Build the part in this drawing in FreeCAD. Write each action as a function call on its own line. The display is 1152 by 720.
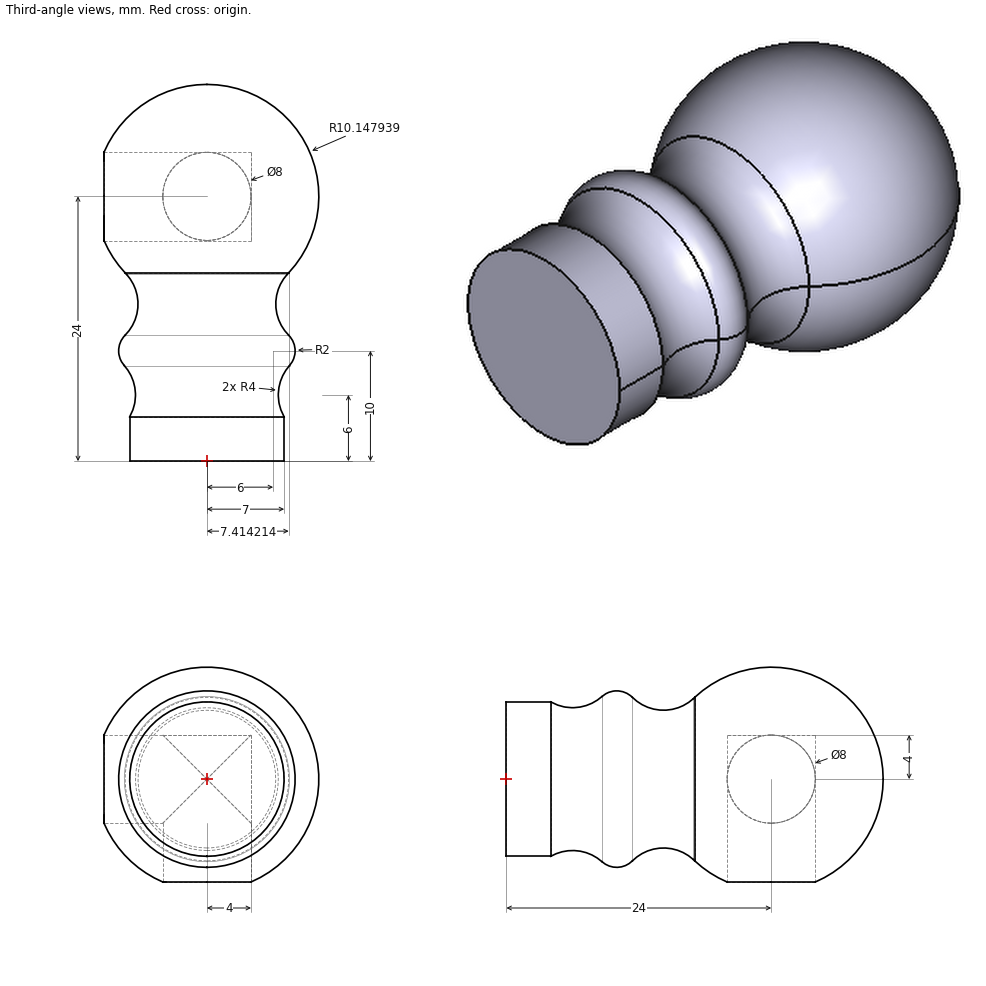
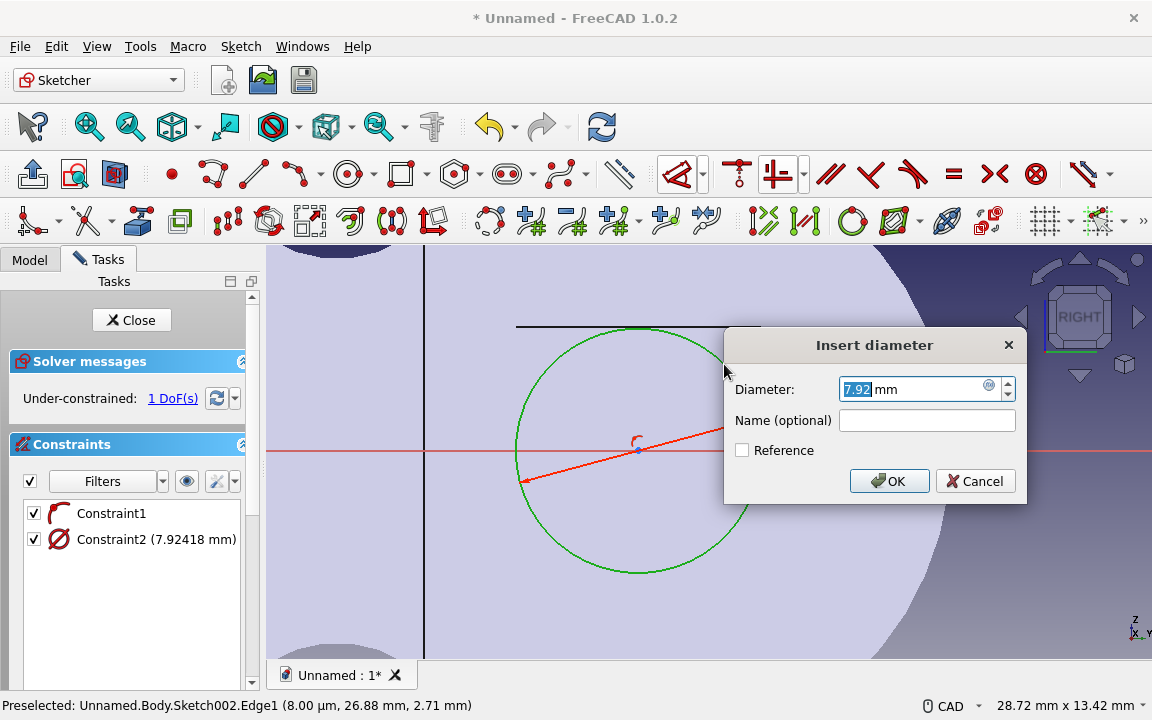
text(8)
key(Return)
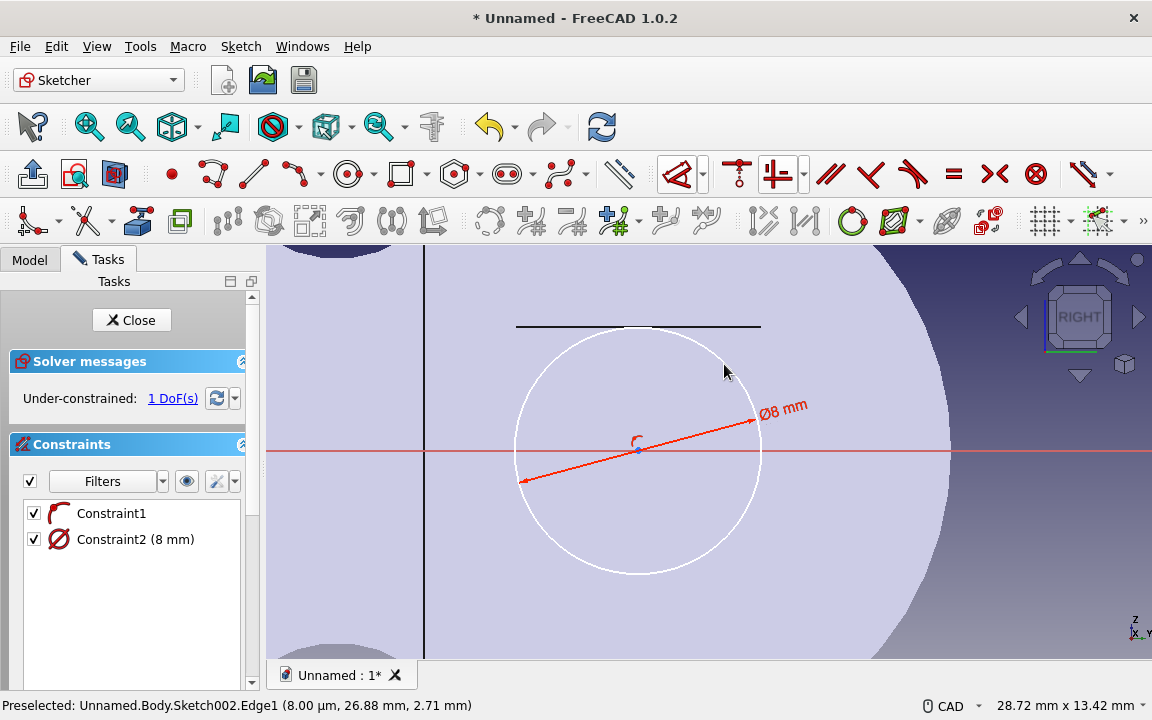
click(638, 451)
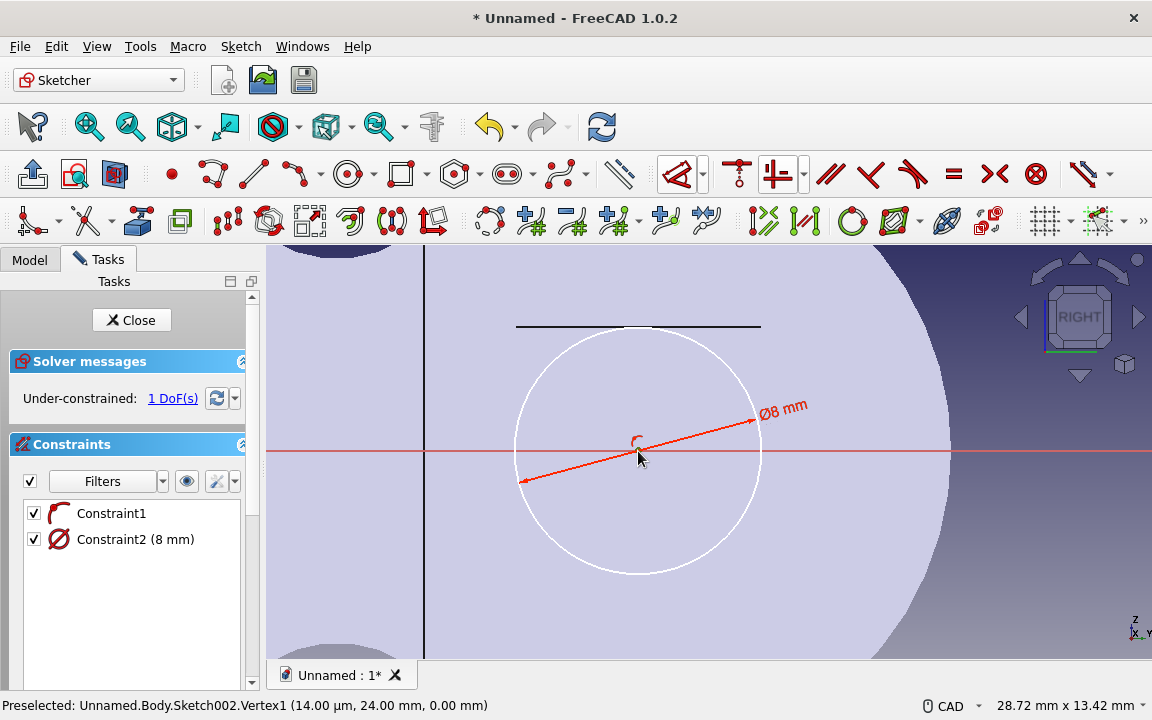
key(l)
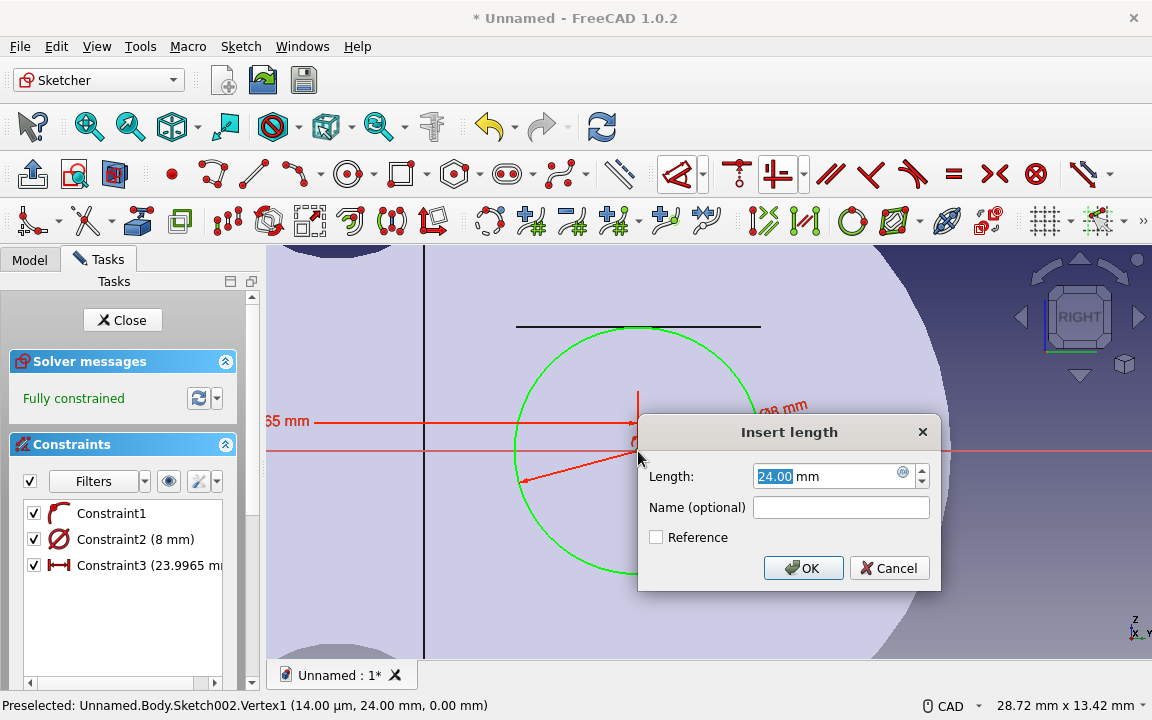
text(24)
key(Return)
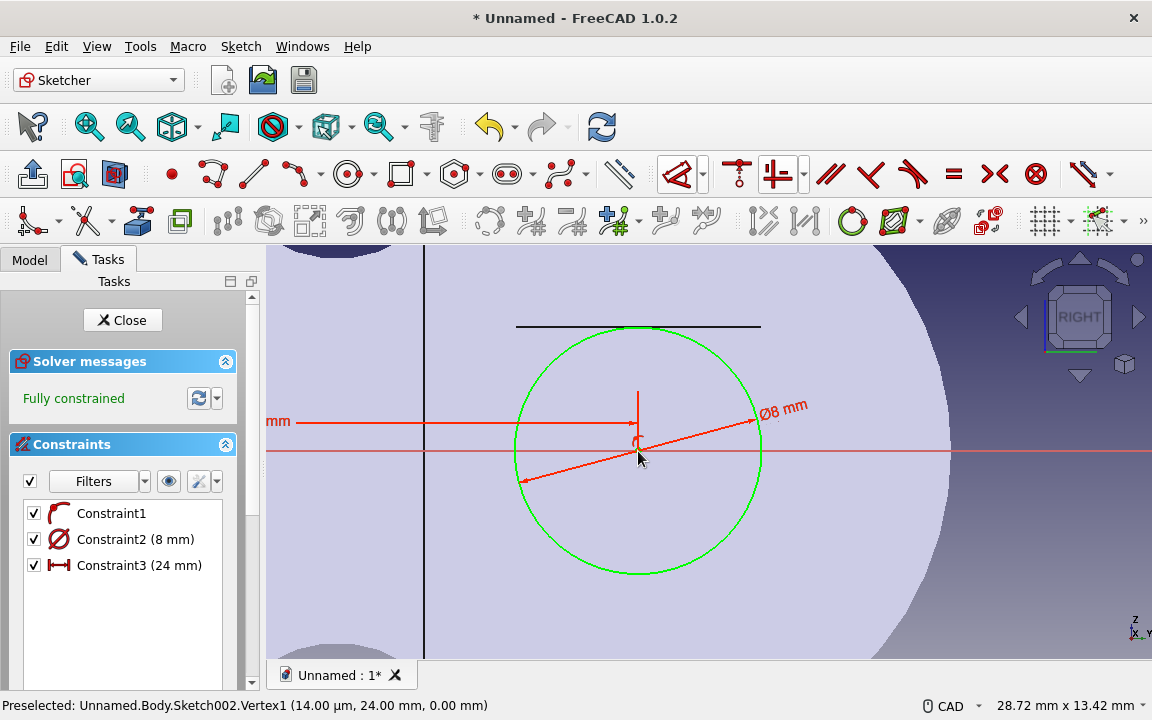
click(123, 320)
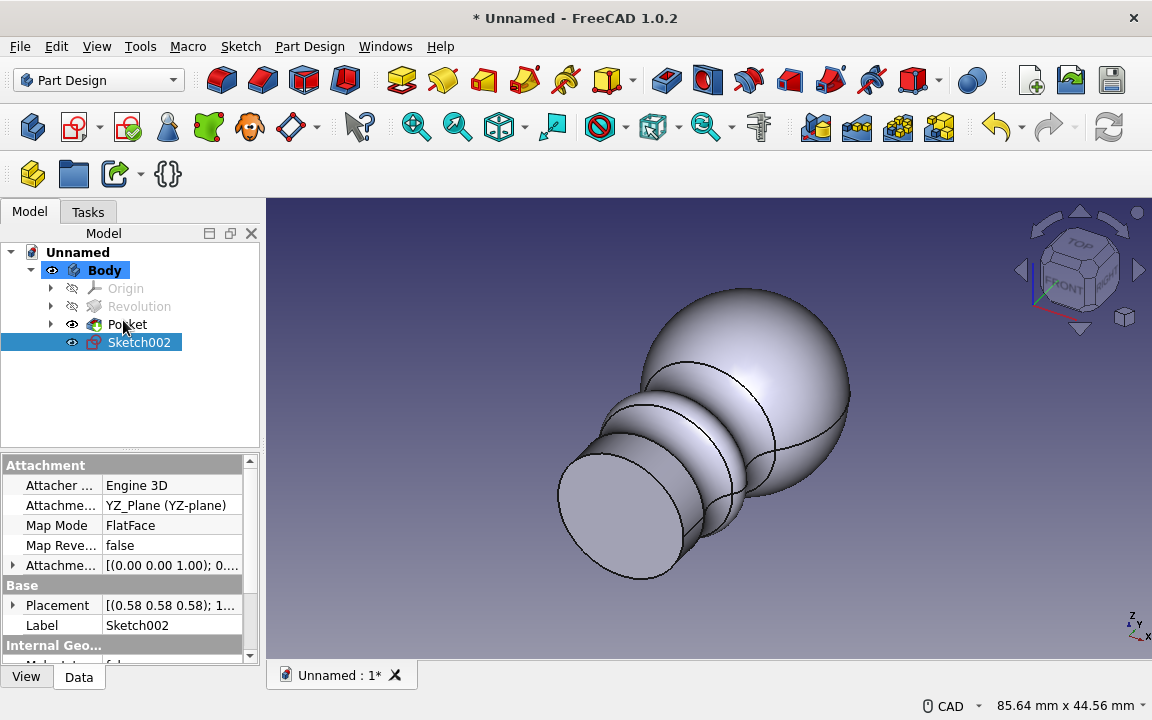
click(667, 80)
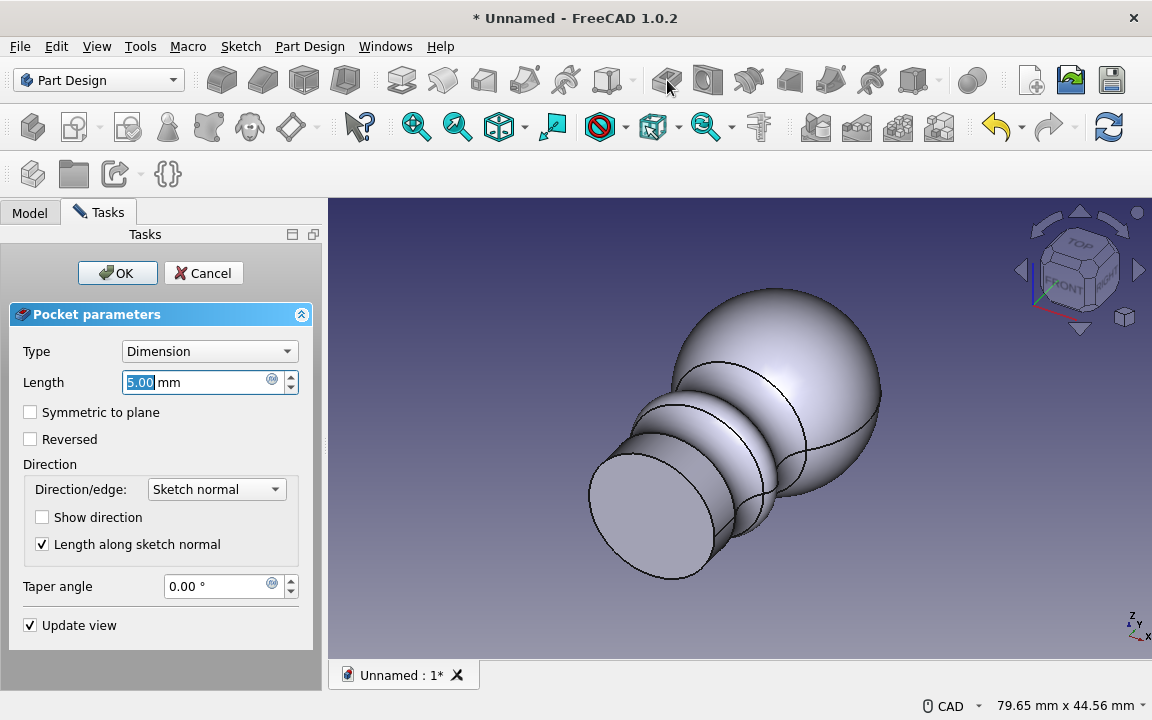
click(210, 352)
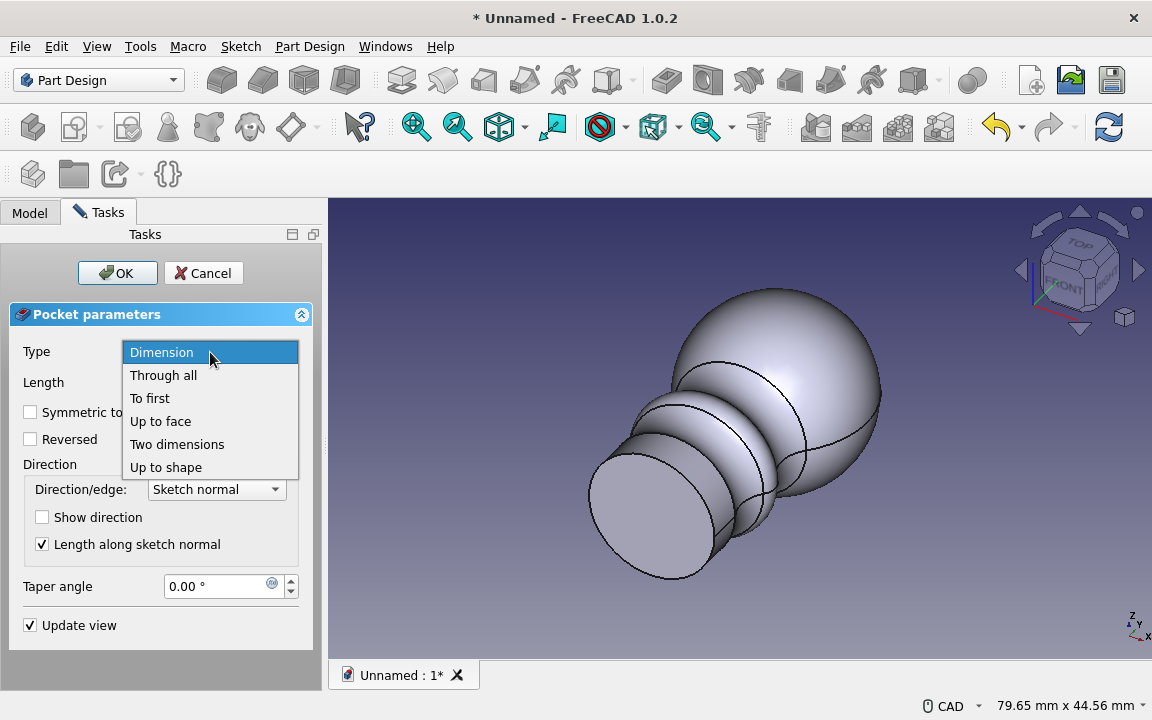
click(208, 444)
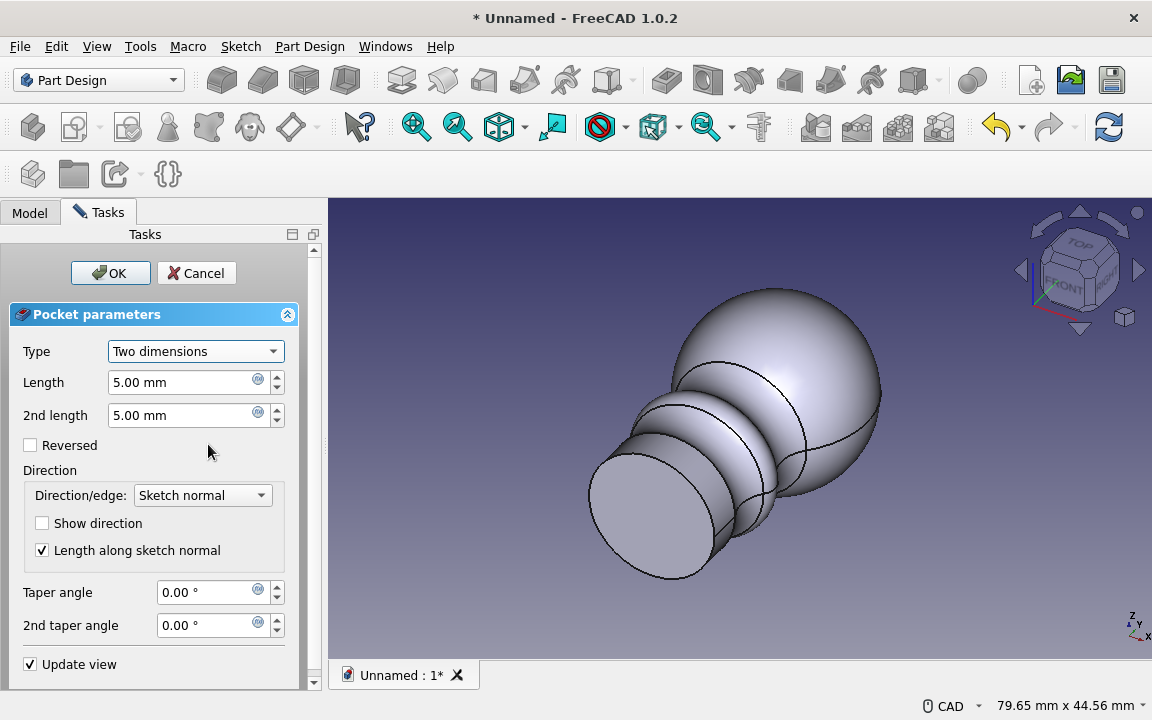
triple_click(190, 382)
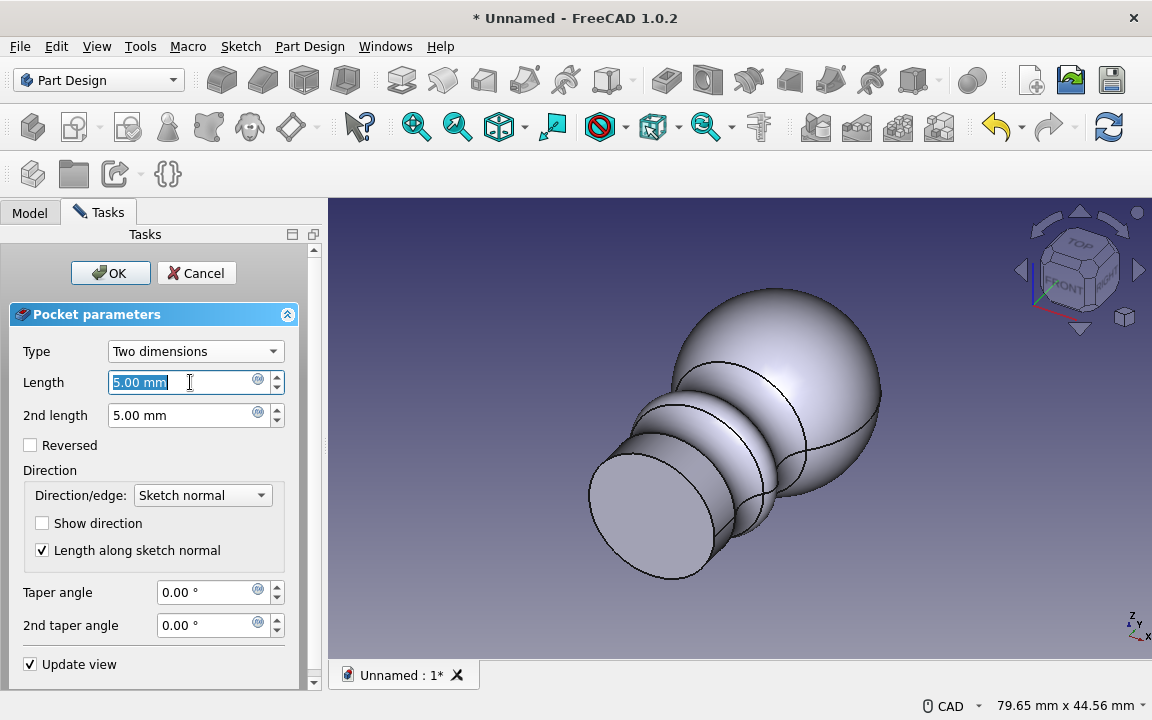
text(4)
key(Tab)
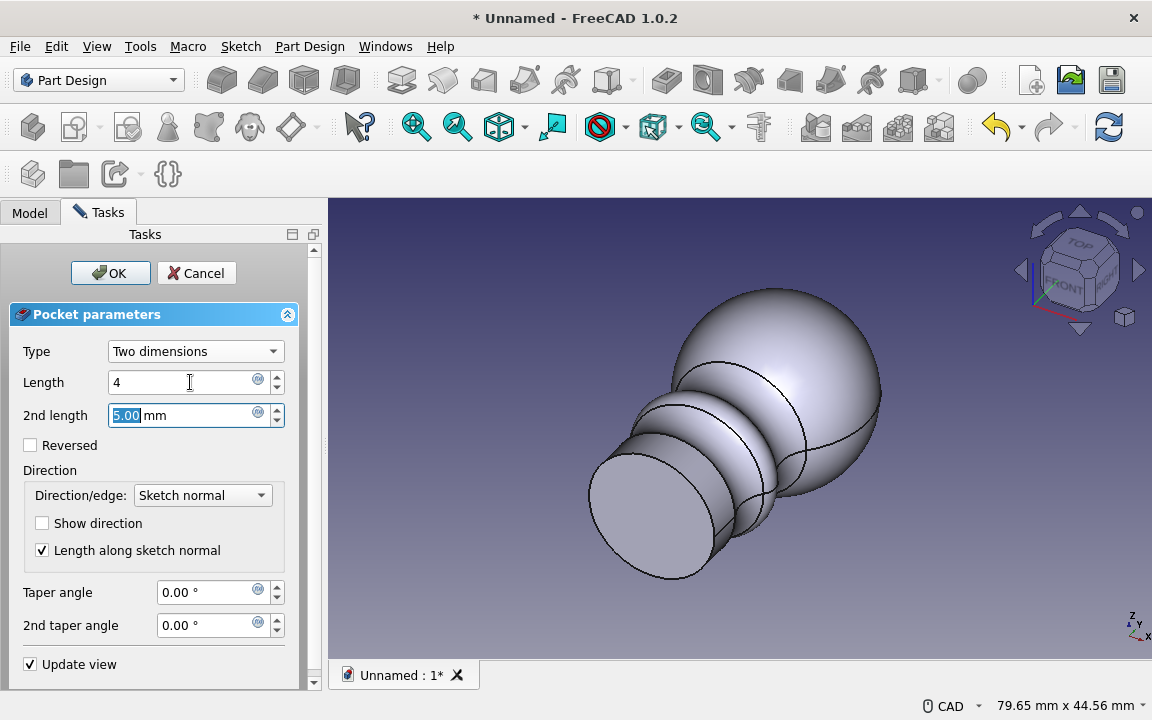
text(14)
key(Tab)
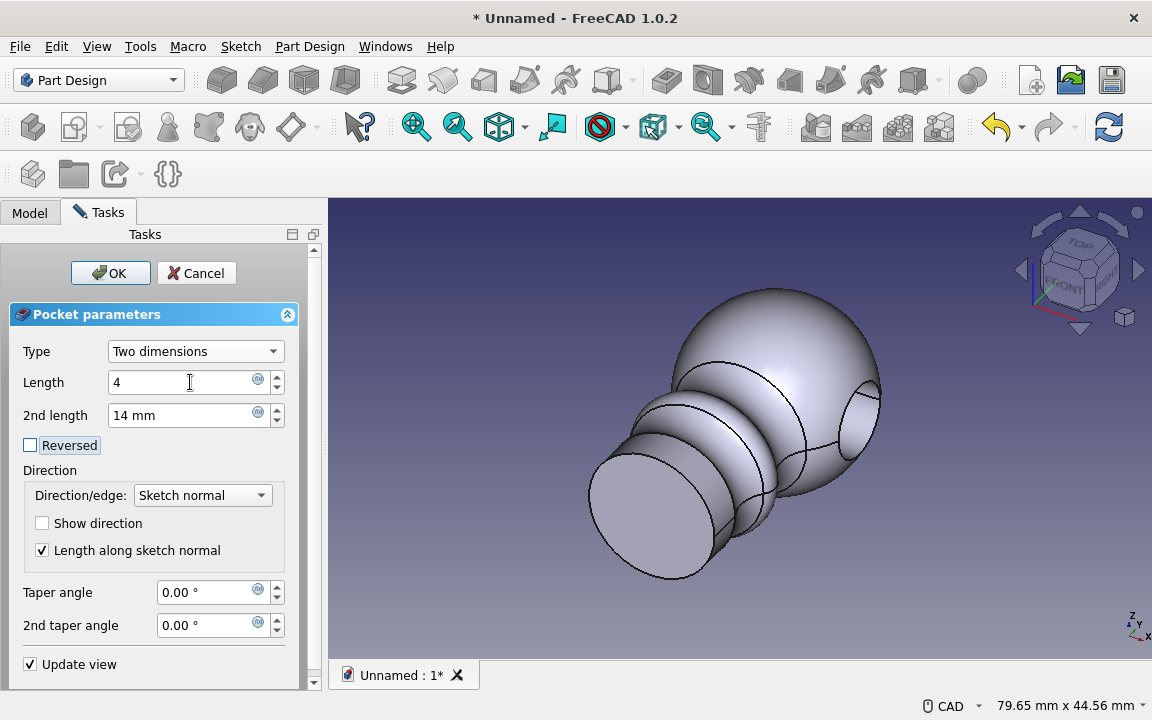
click(31, 445)